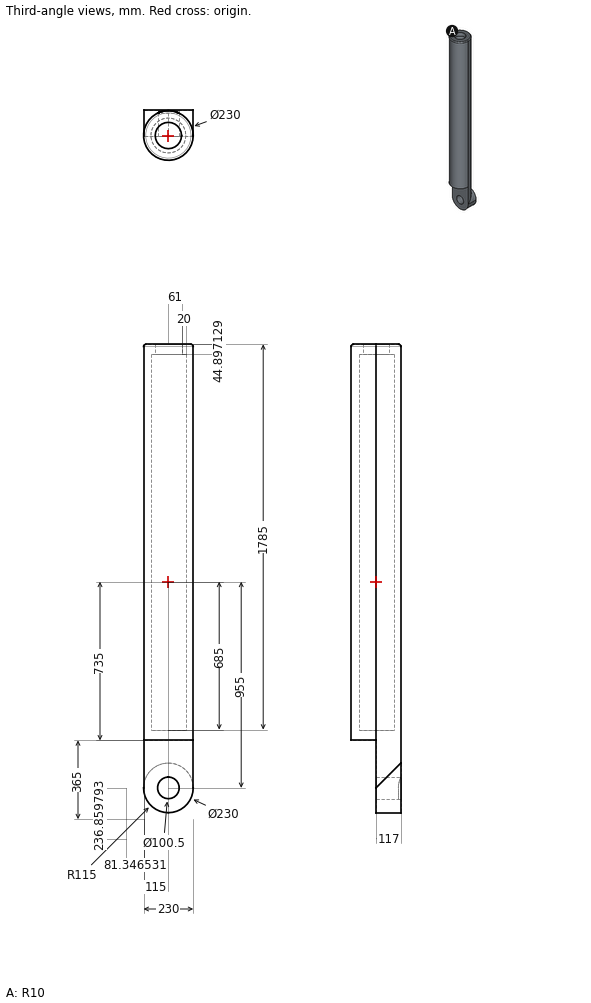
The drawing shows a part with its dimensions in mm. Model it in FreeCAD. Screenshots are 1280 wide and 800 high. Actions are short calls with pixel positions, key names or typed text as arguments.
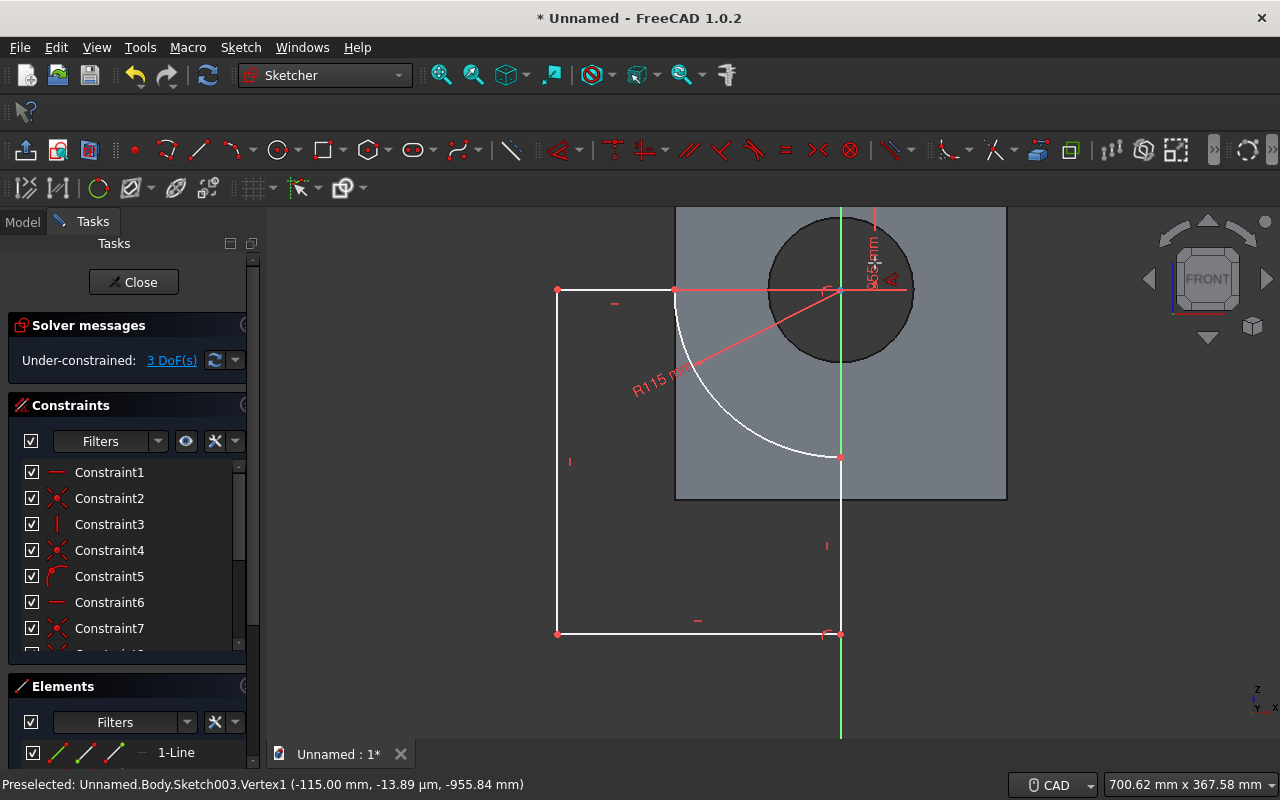
click(841, 291)
click(783, 263)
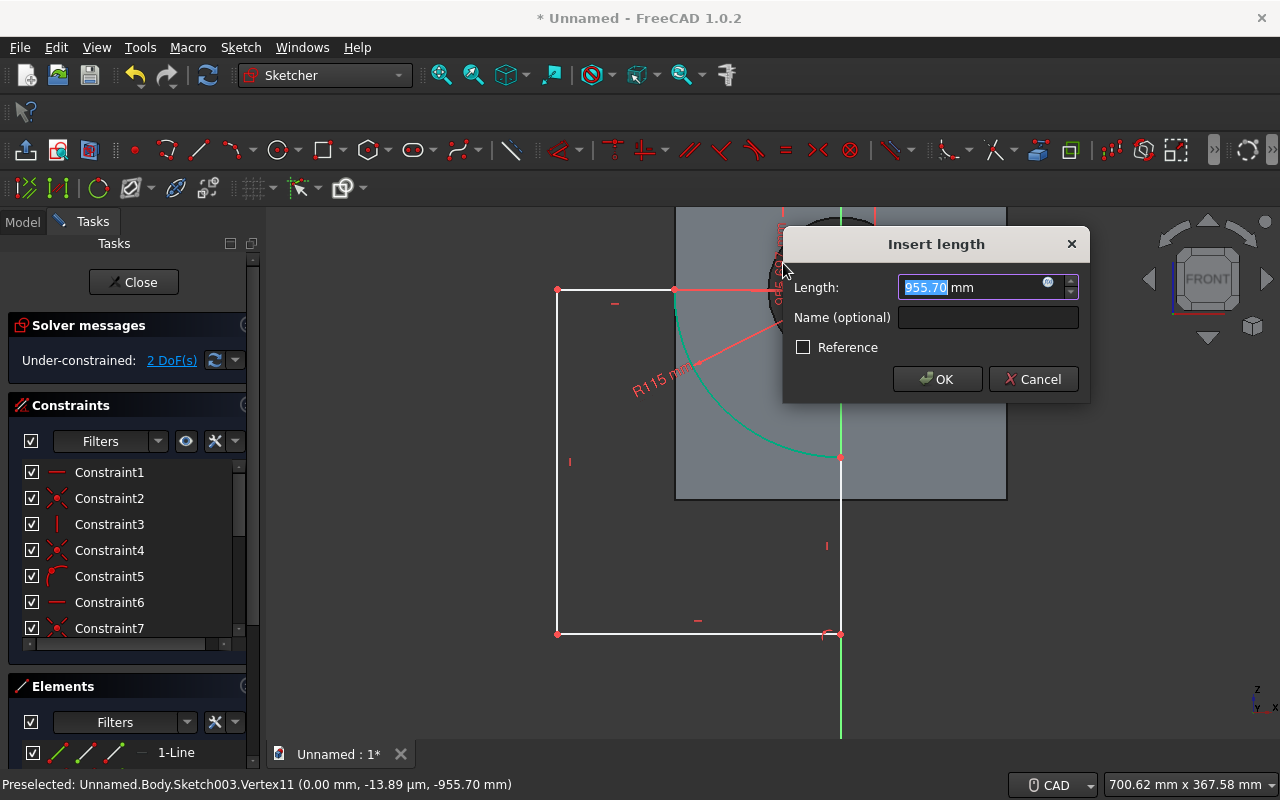
text(955)
key(Return)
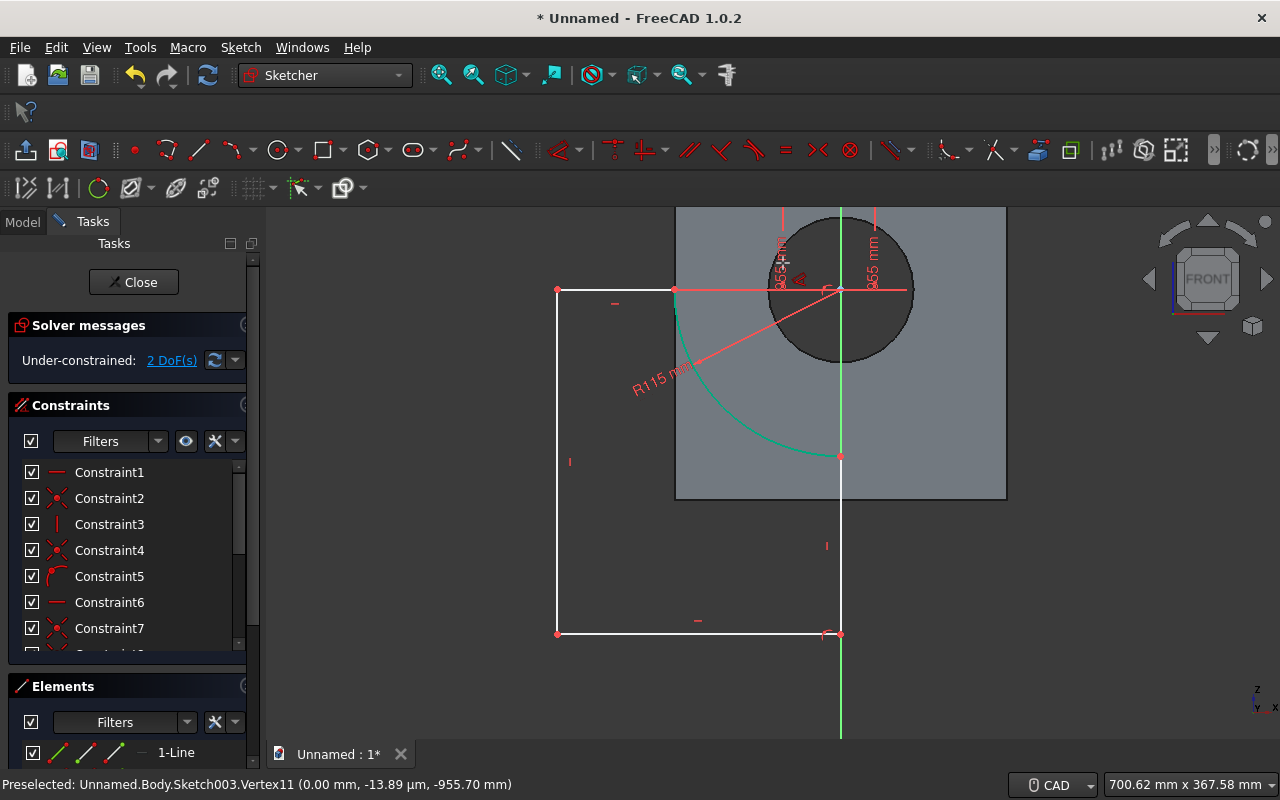
click(639, 290)
click(616, 256)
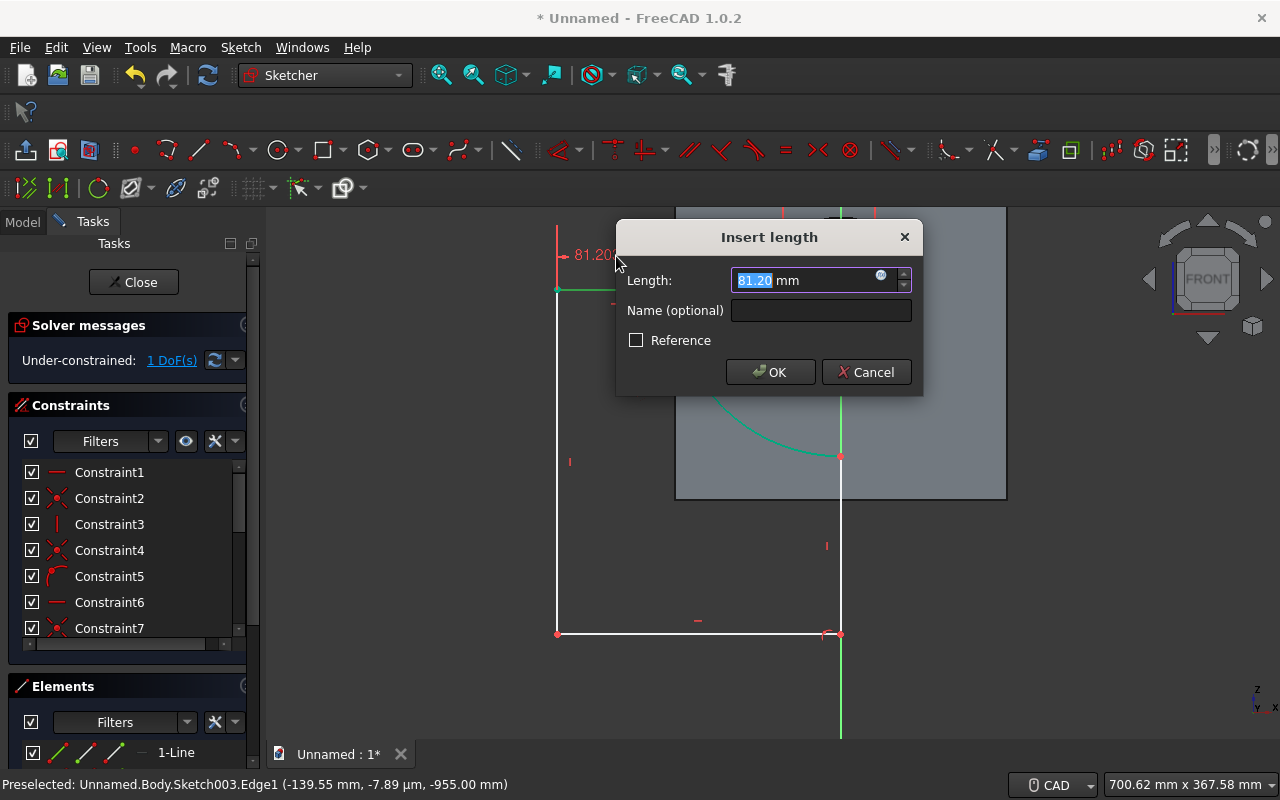
text(81.346531)
key(Return)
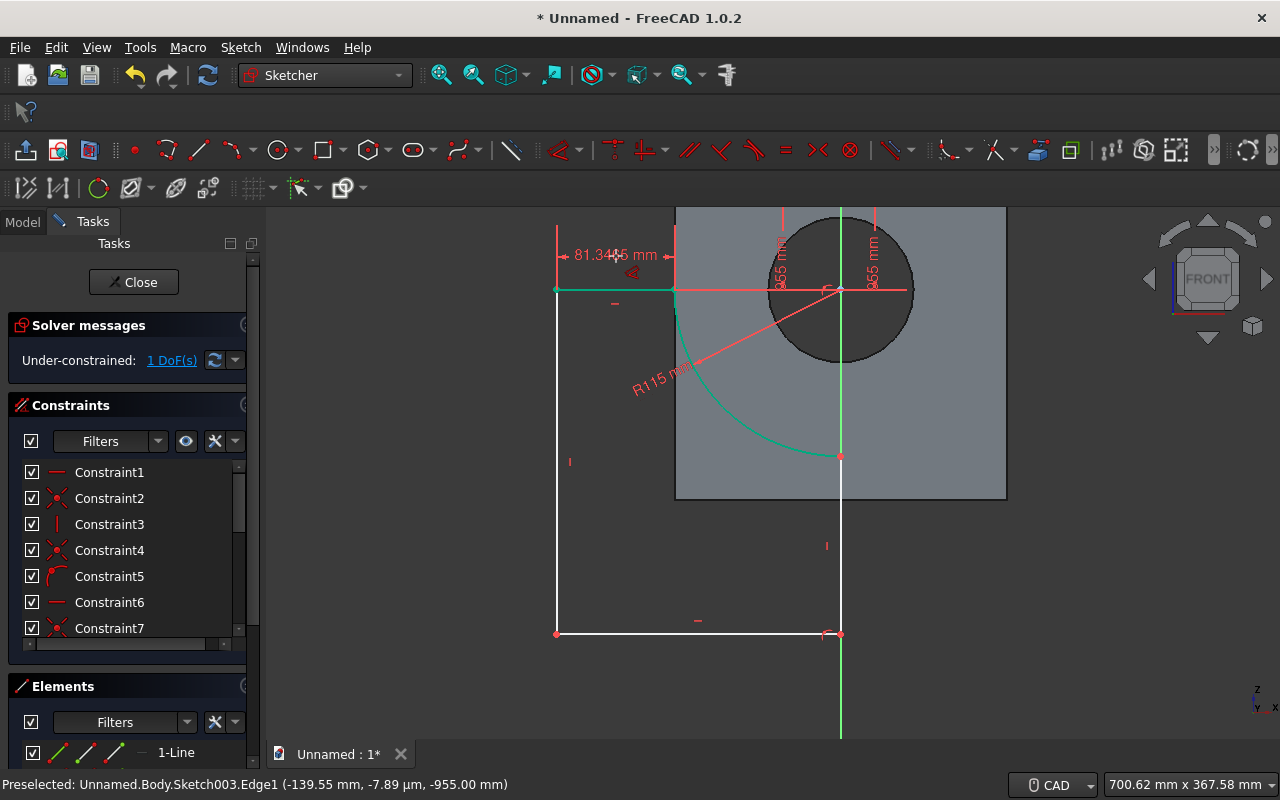
click(557, 393)
click(523, 462)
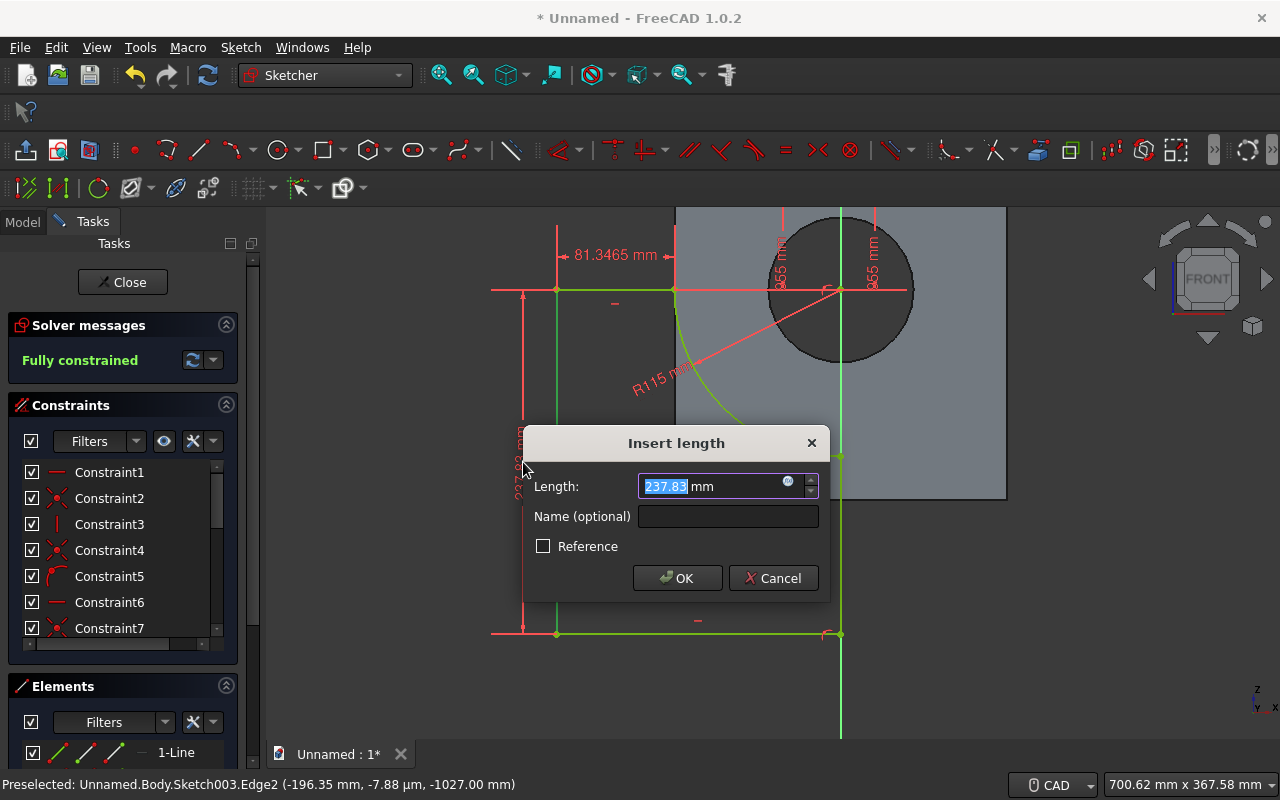
text(236.859793)
key(Return)
key(Escape)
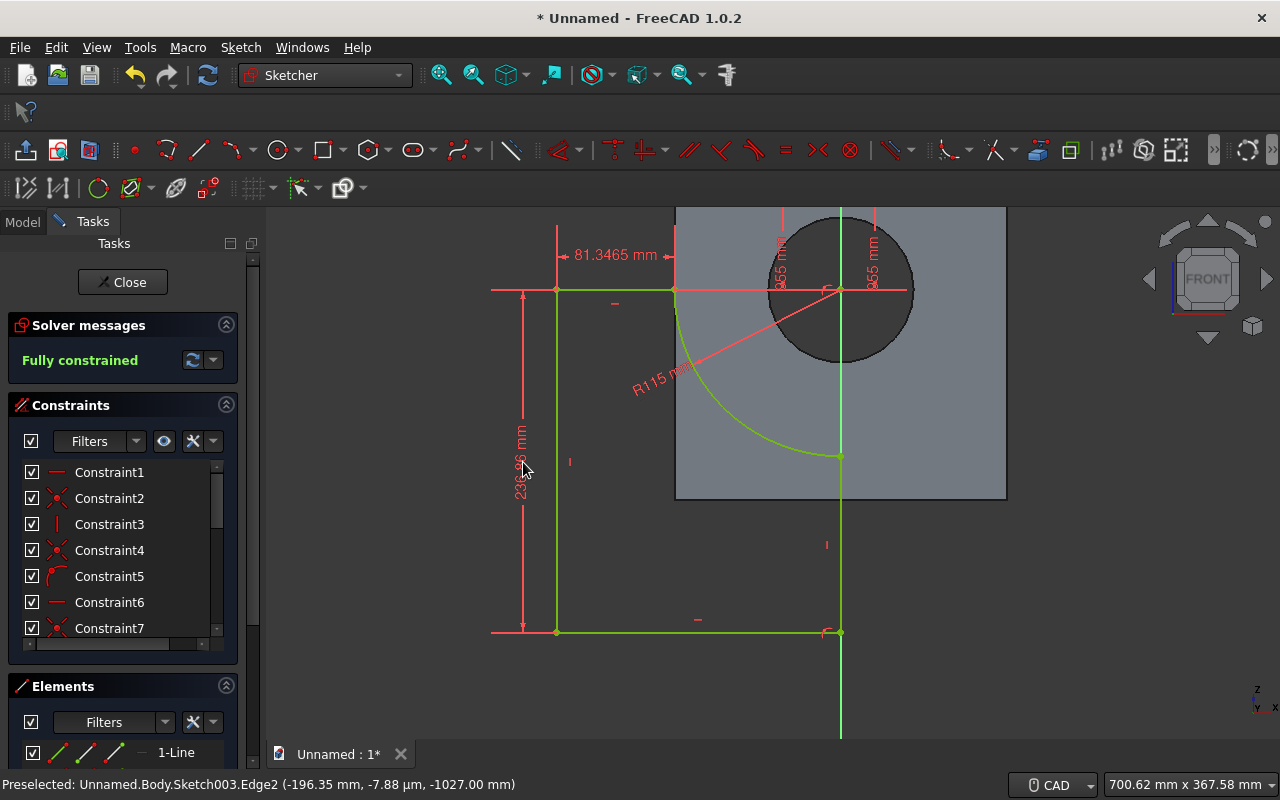
click(123, 282)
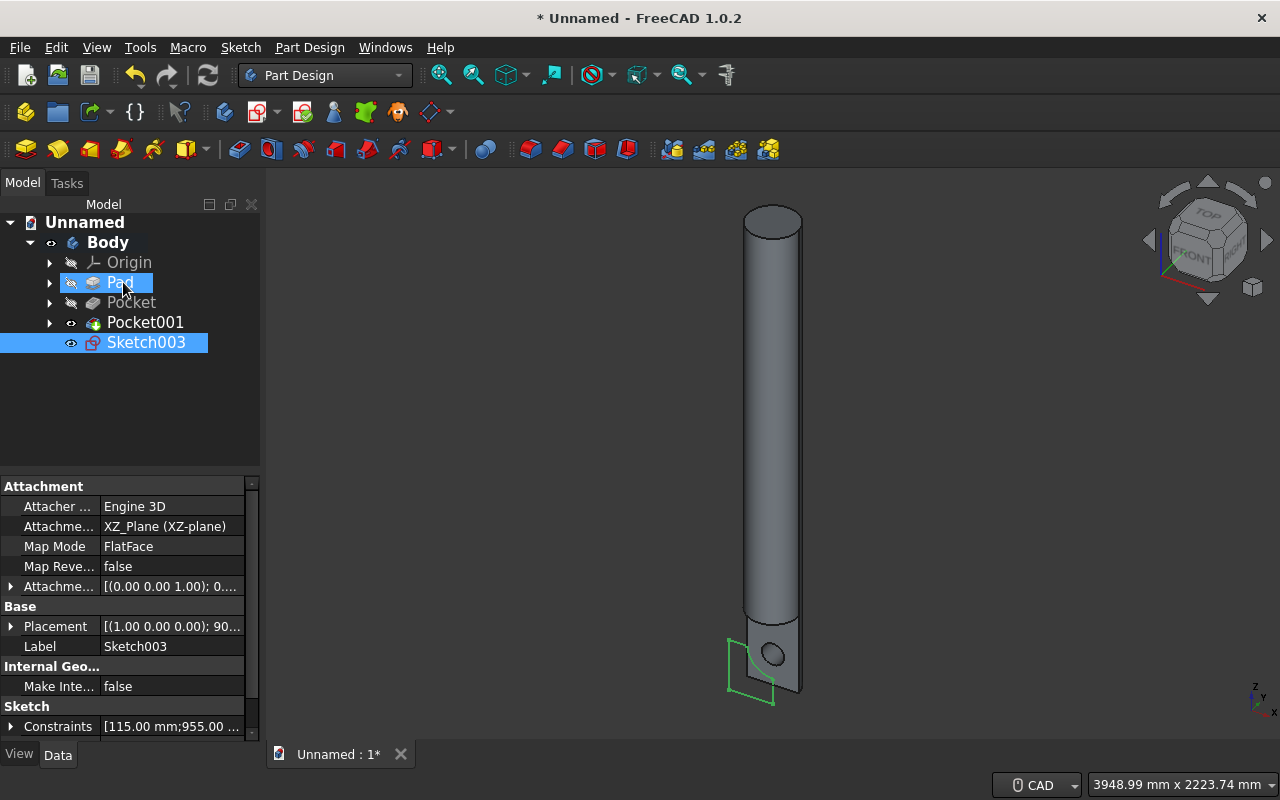
click(304, 150)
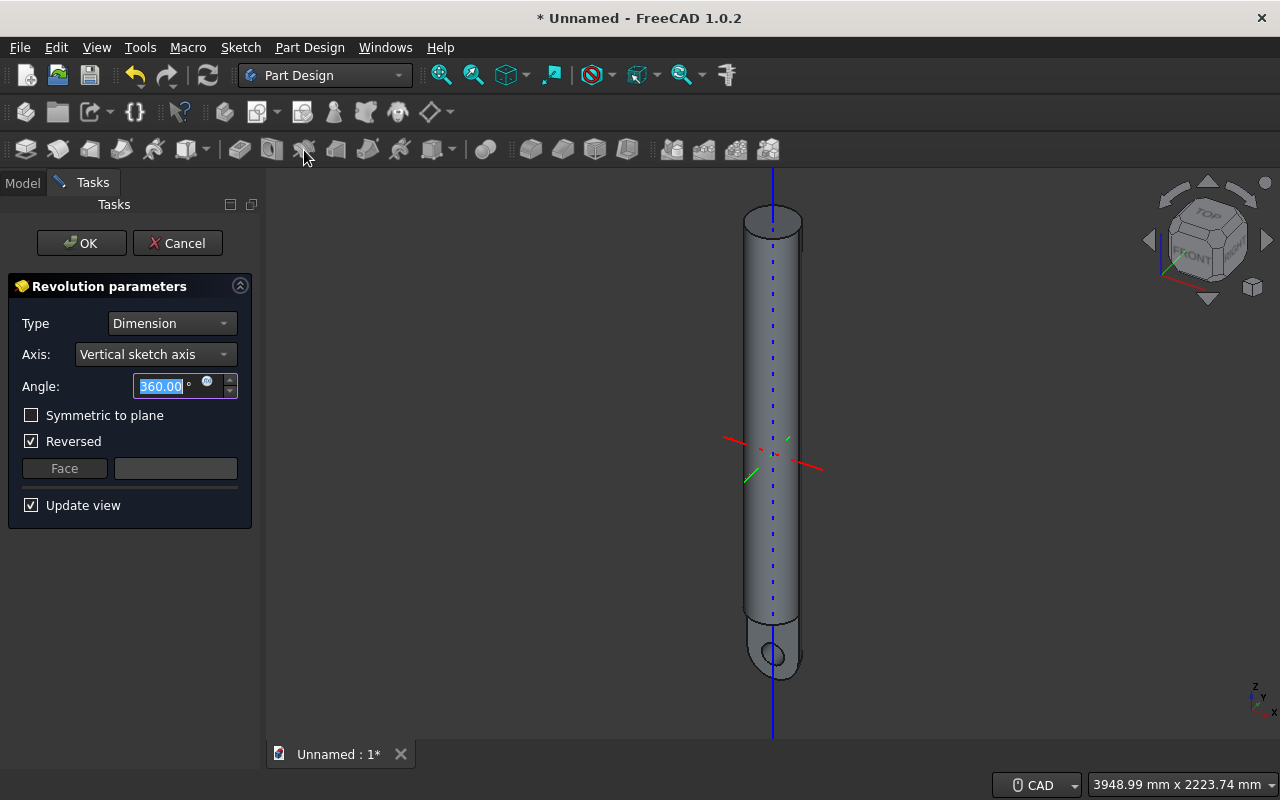
click(82, 243)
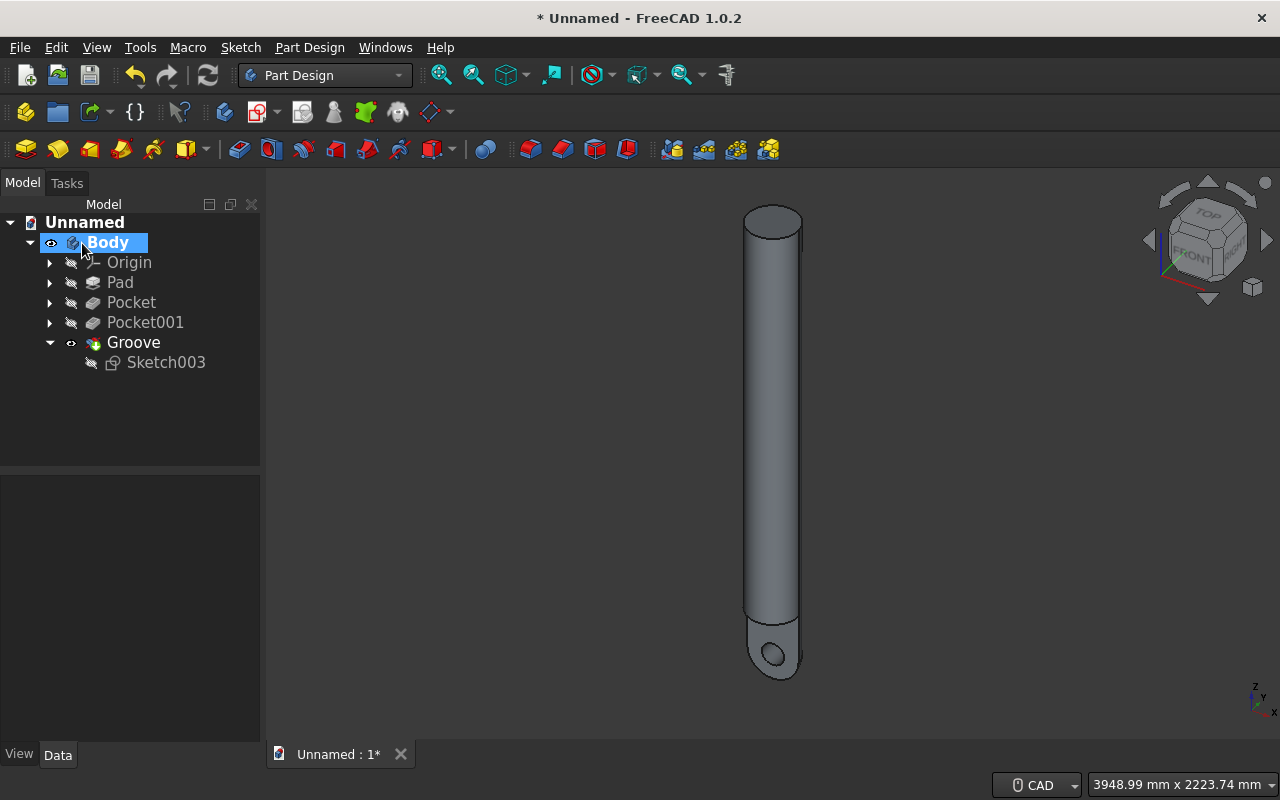
click(780, 635)